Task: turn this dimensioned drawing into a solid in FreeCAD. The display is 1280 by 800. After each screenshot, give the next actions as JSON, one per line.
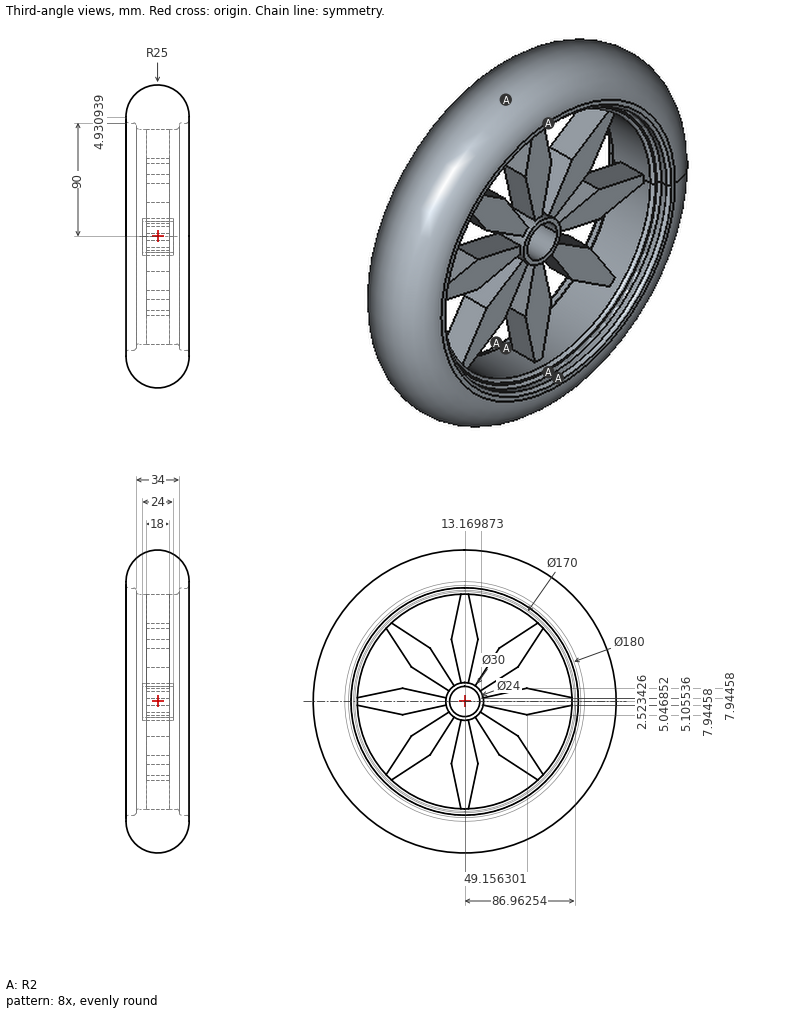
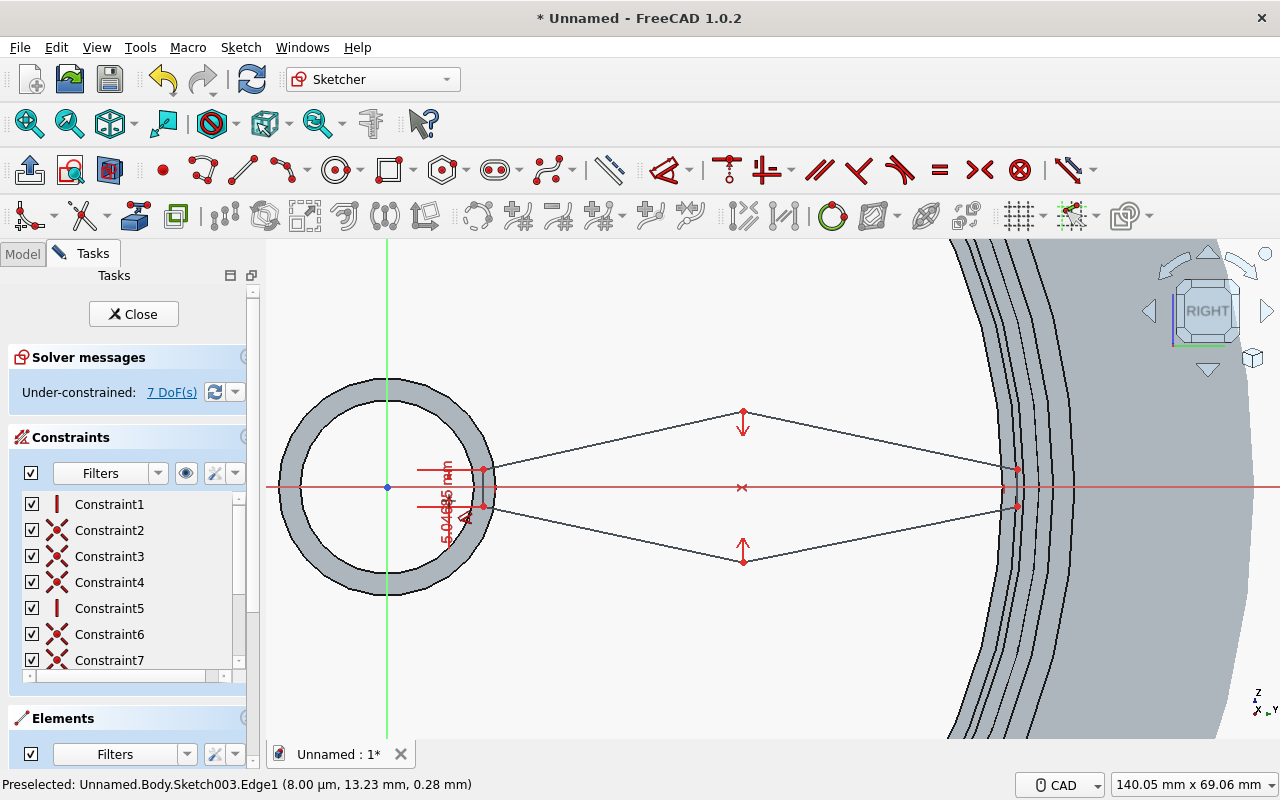
{"action": "left_click", "coordinate": [1017, 485]}
{"action": "left_click", "coordinate": [1051, 501]}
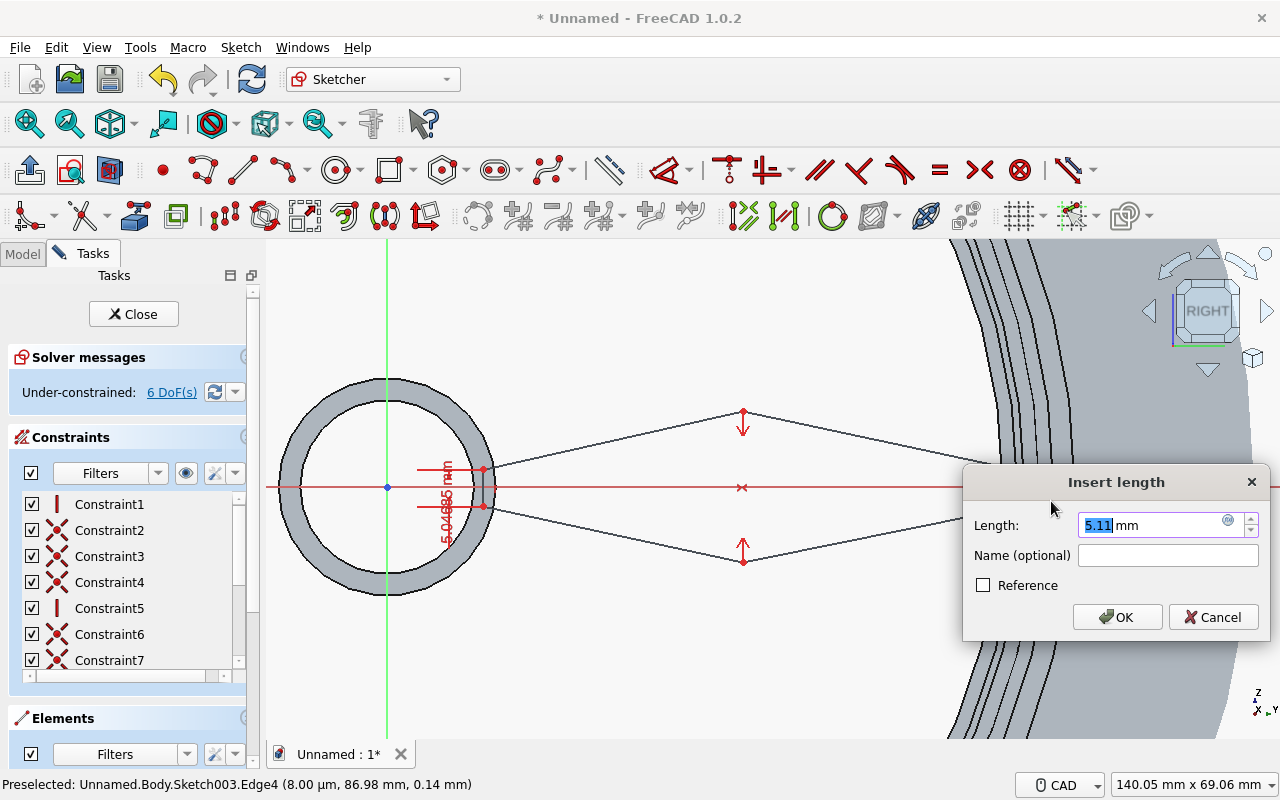
{"action": "type", "text": "5.105536"}
{"action": "key", "text": "Return"}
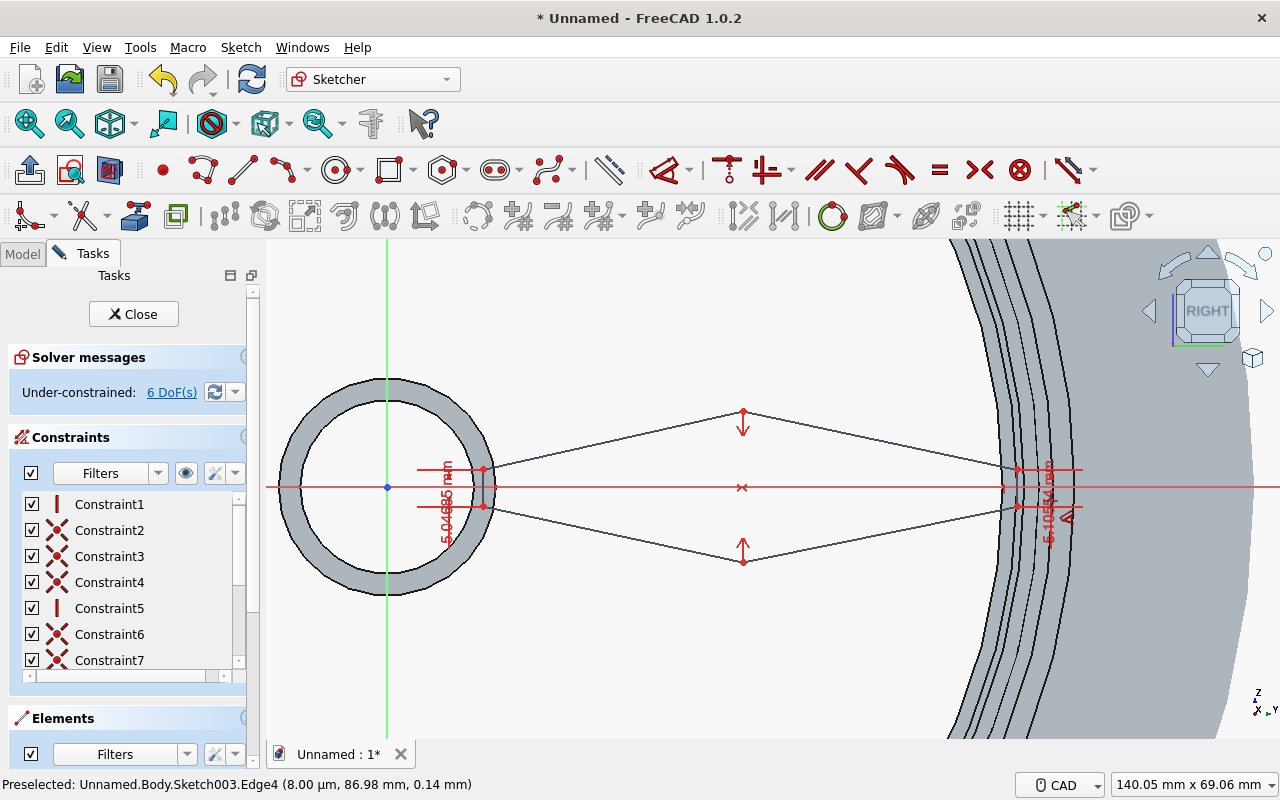
{"action": "left_click", "coordinate": [825, 546]}
{"action": "left_click", "coordinate": [1051, 535]}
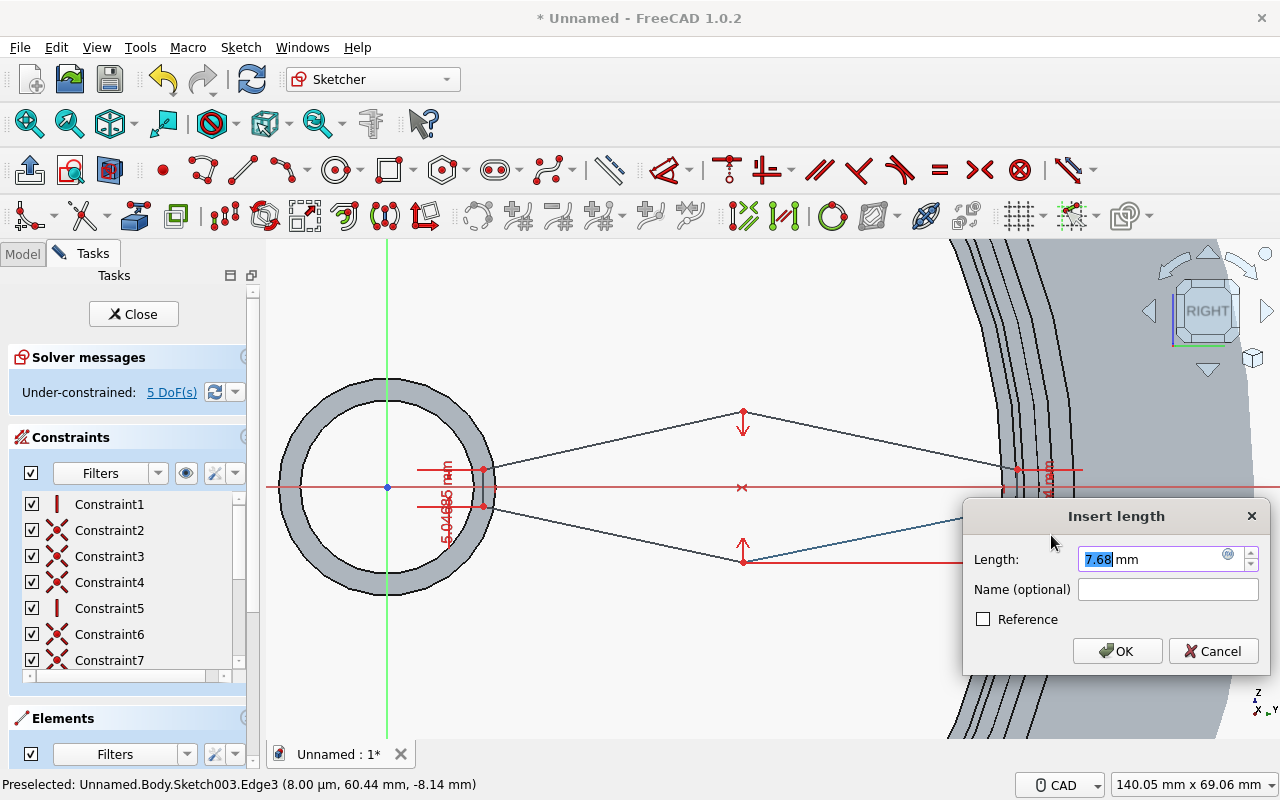
{"action": "type", "text": "7.94458"}
{"action": "key", "text": "Return"}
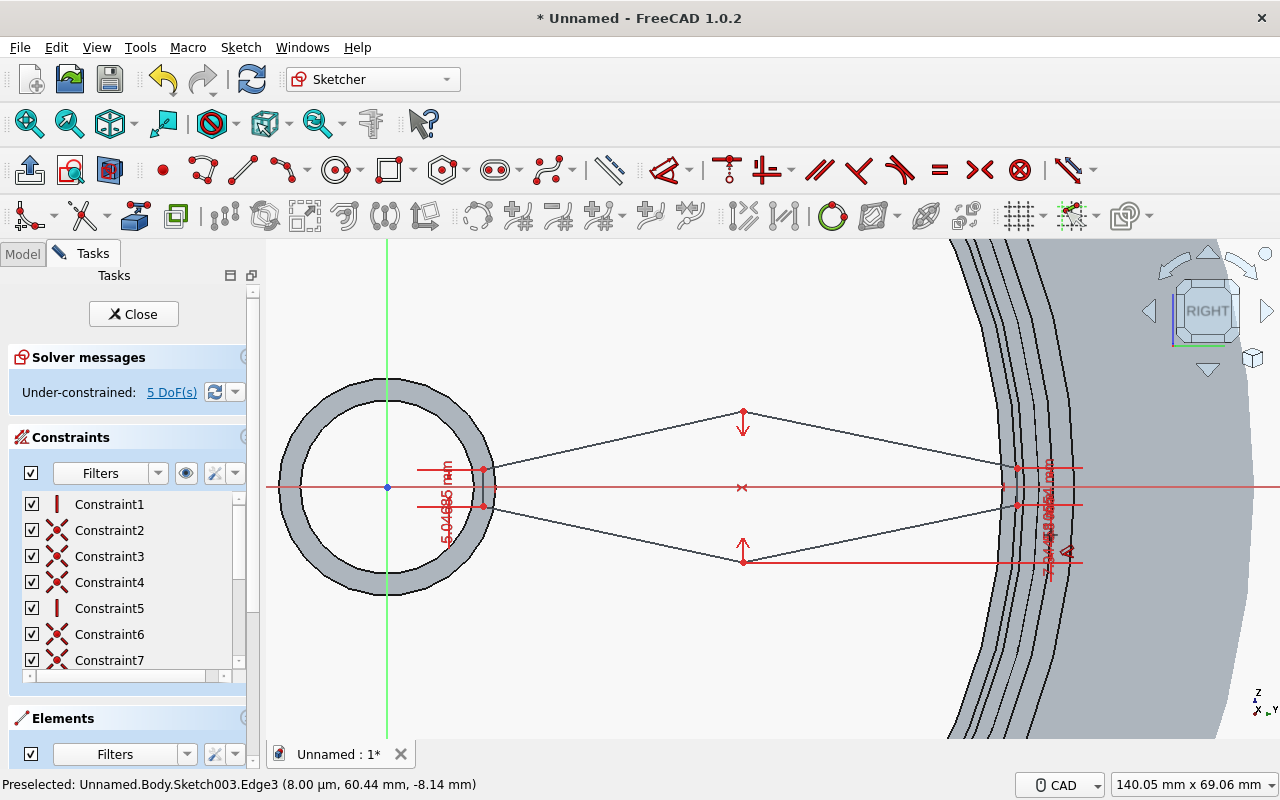
{"action": "left_click", "coordinate": [935, 451]}
{"action": "left_click", "coordinate": [1051, 440]}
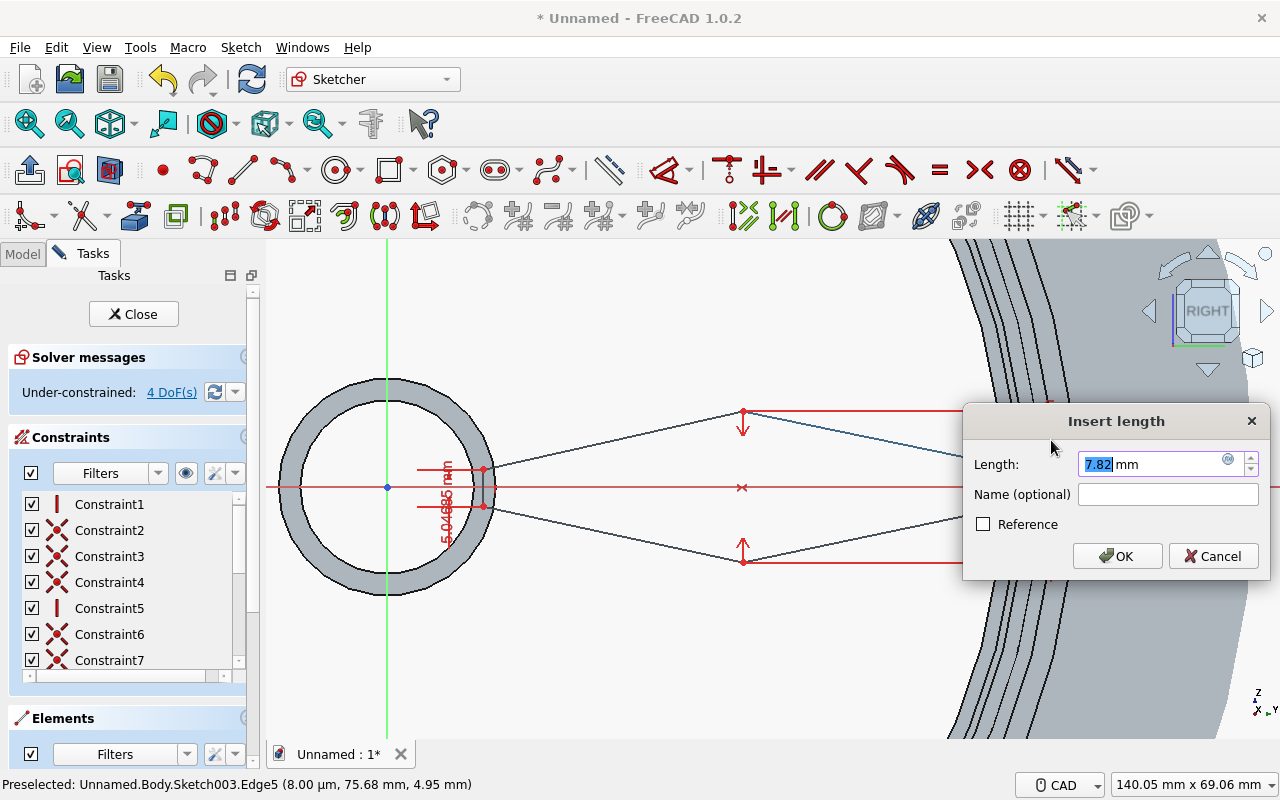
{"action": "type", "text": "7.94458"}
{"action": "key", "text": "Return"}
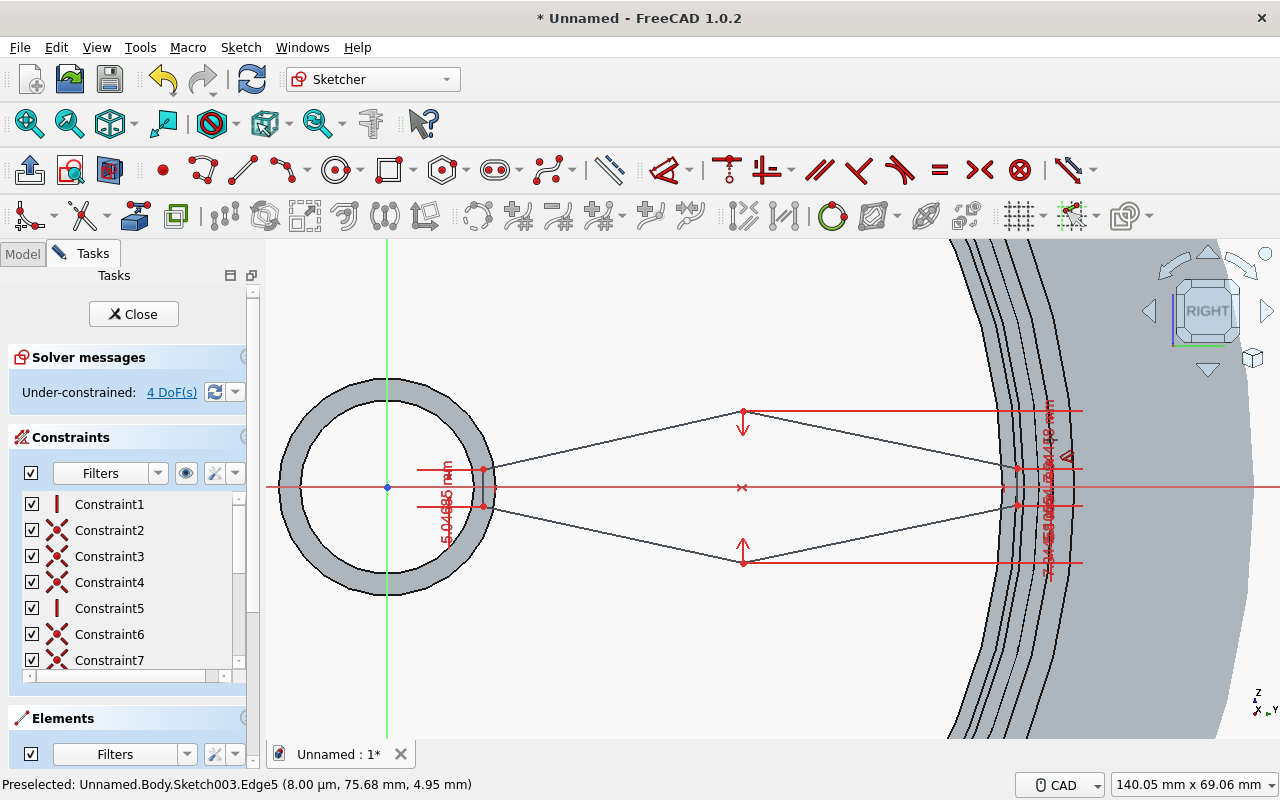
{"action": "scroll", "coordinate": [483, 470], "scroll_direction": "up", "scroll_amount": 4}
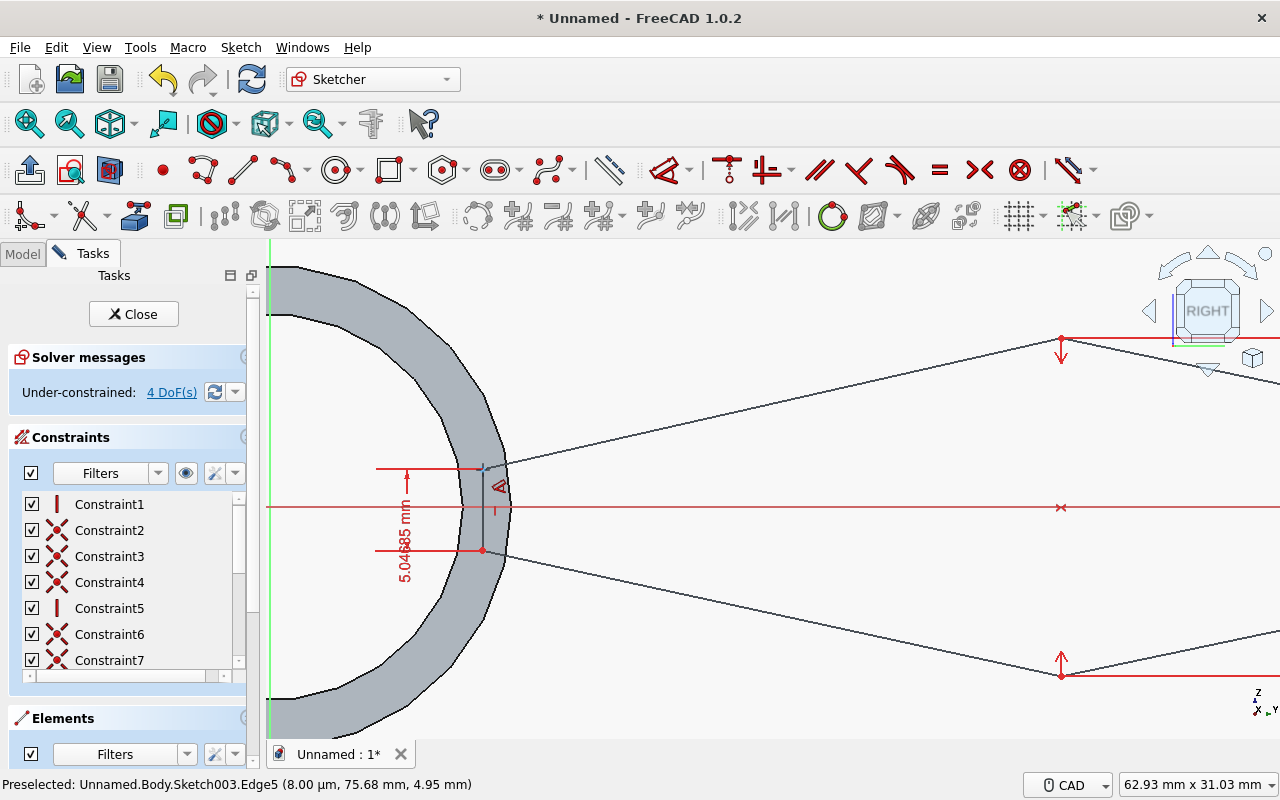
{"action": "left_click", "coordinate": [483, 469]}
{"action": "left_click", "coordinate": [517, 488]}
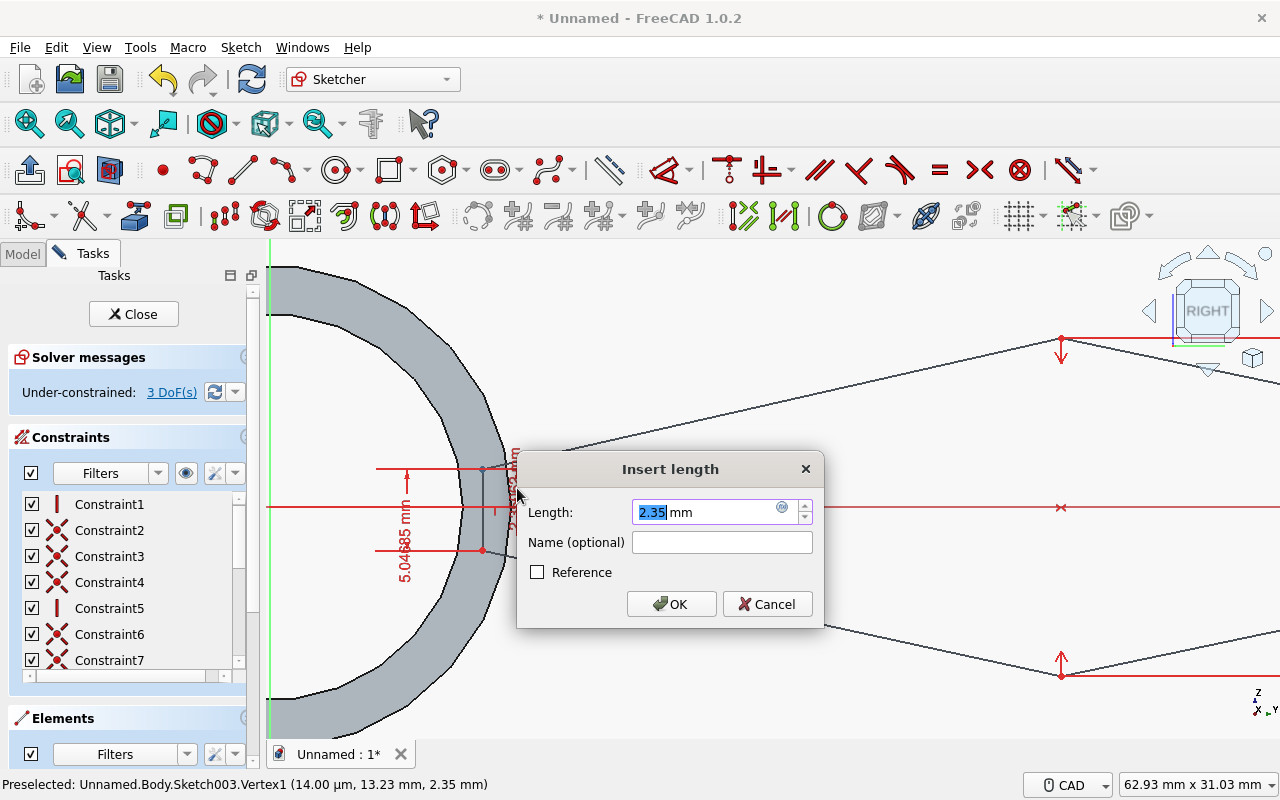
{"action": "type", "text": "2.523426"}
{"action": "key", "text": "Return"}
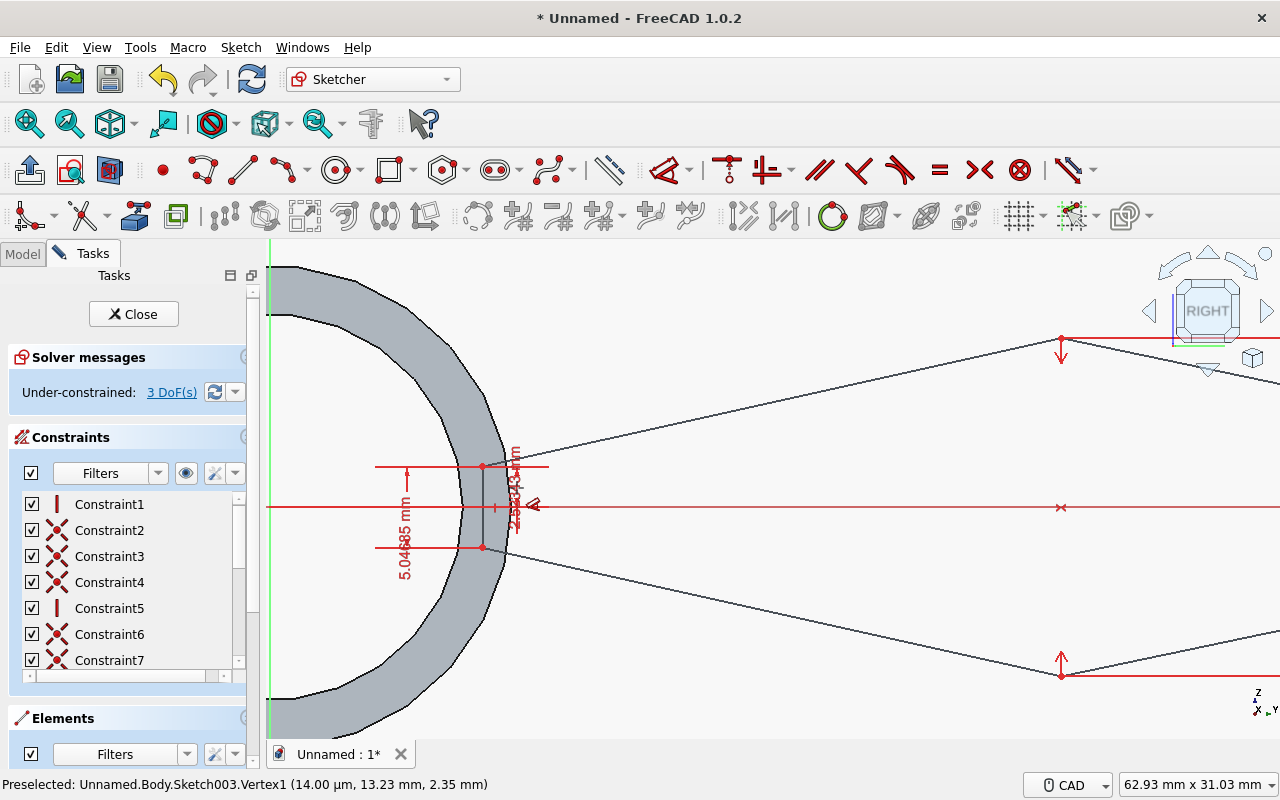
{"action": "scroll", "coordinate": [488, 474], "scroll_direction": "down", "scroll_amount": 4}